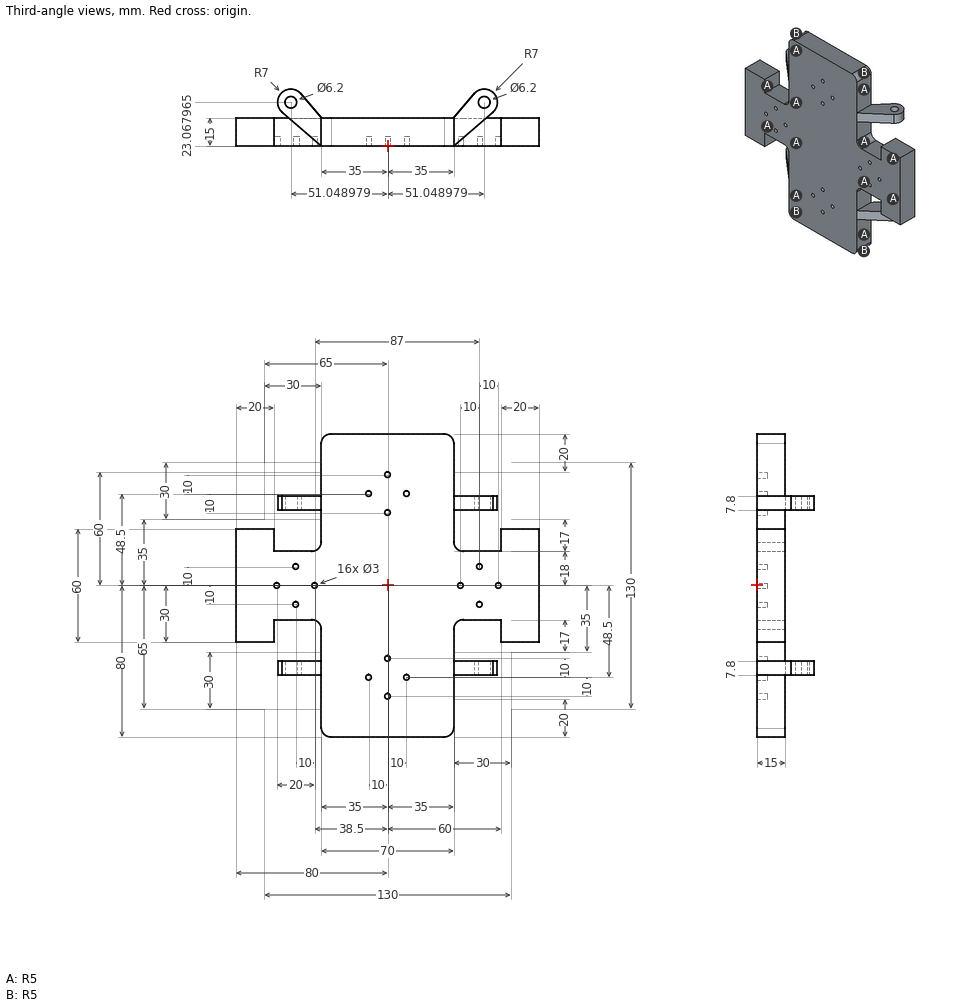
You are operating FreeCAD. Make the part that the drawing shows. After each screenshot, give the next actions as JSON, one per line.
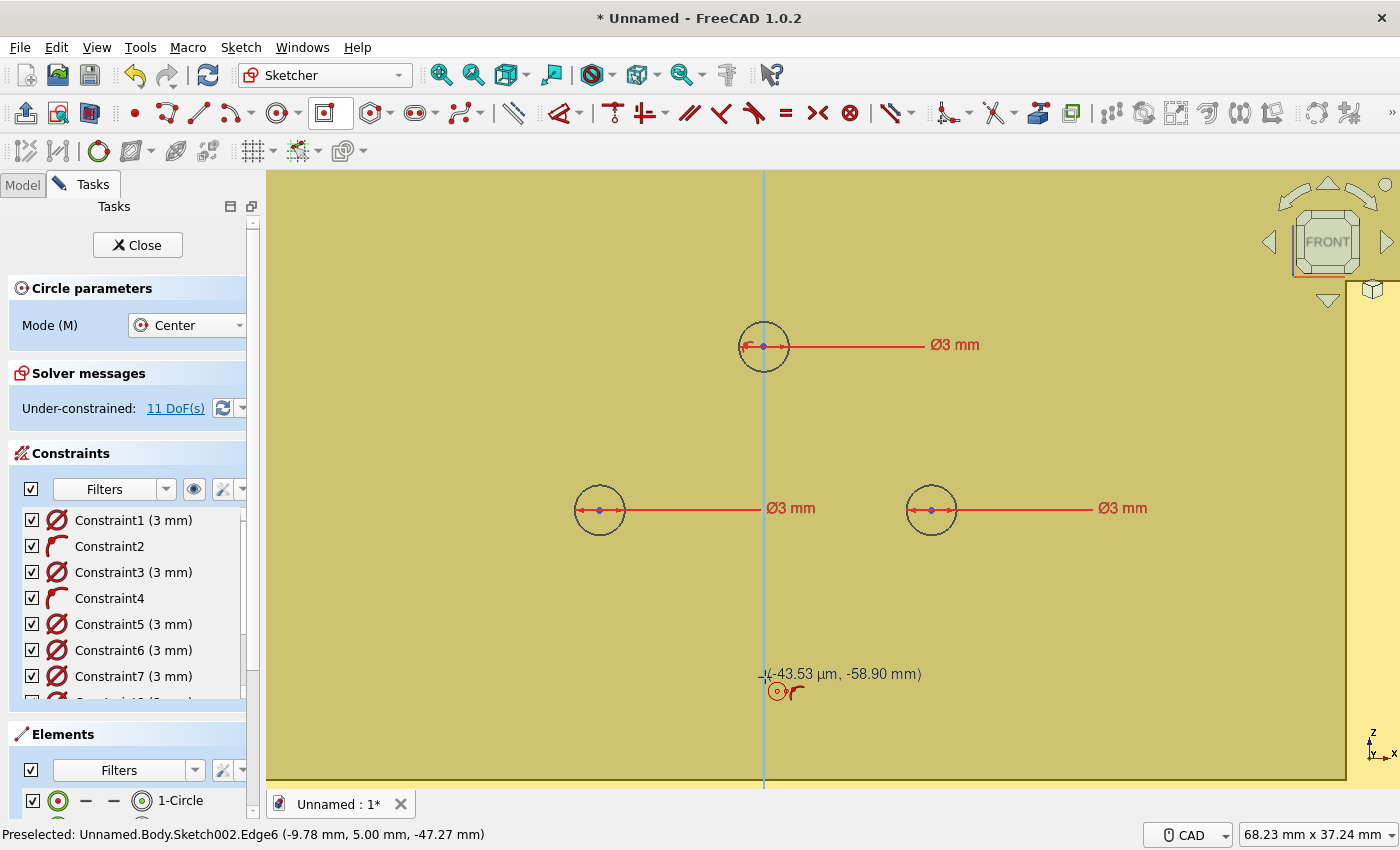
{"action": "scroll", "coordinate": [765, 677], "scroll_direction": "down", "scroll_amount": 8}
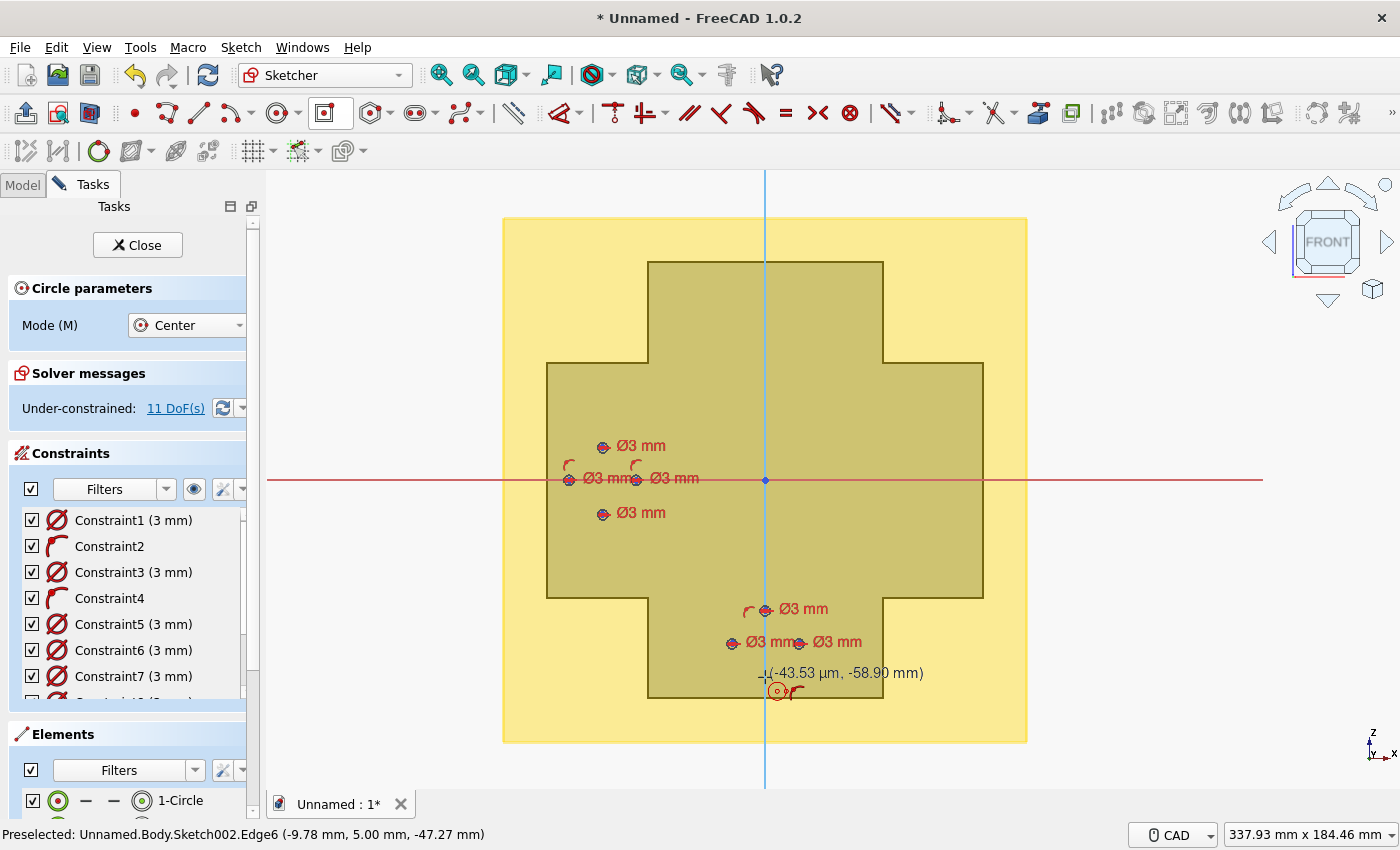
{"action": "left_click", "coordinate": [765, 677]}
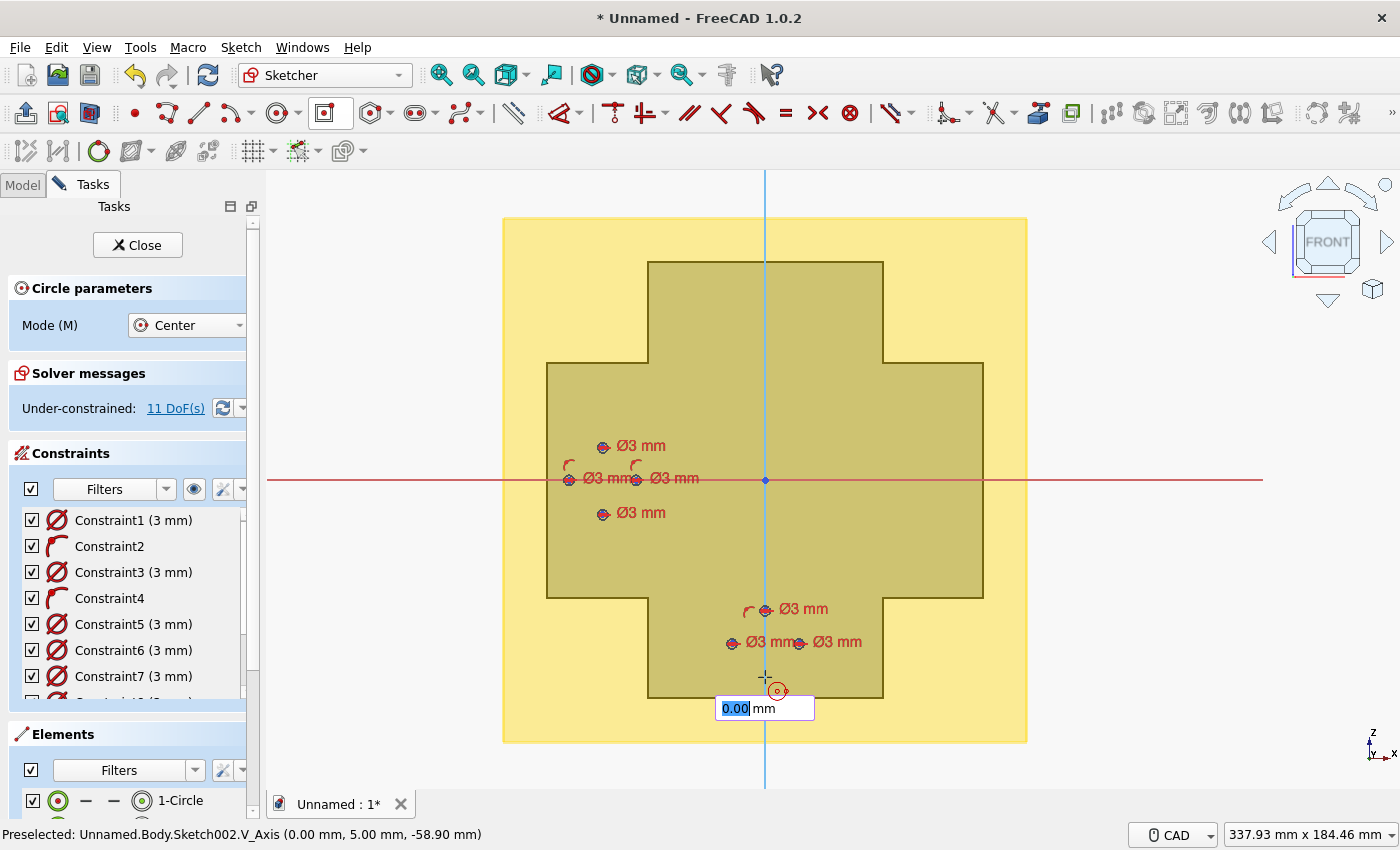
{"action": "scroll", "coordinate": [770, 675], "scroll_direction": "up", "scroll_amount": 7}
{"action": "mouse_move", "coordinate": [768, 672]}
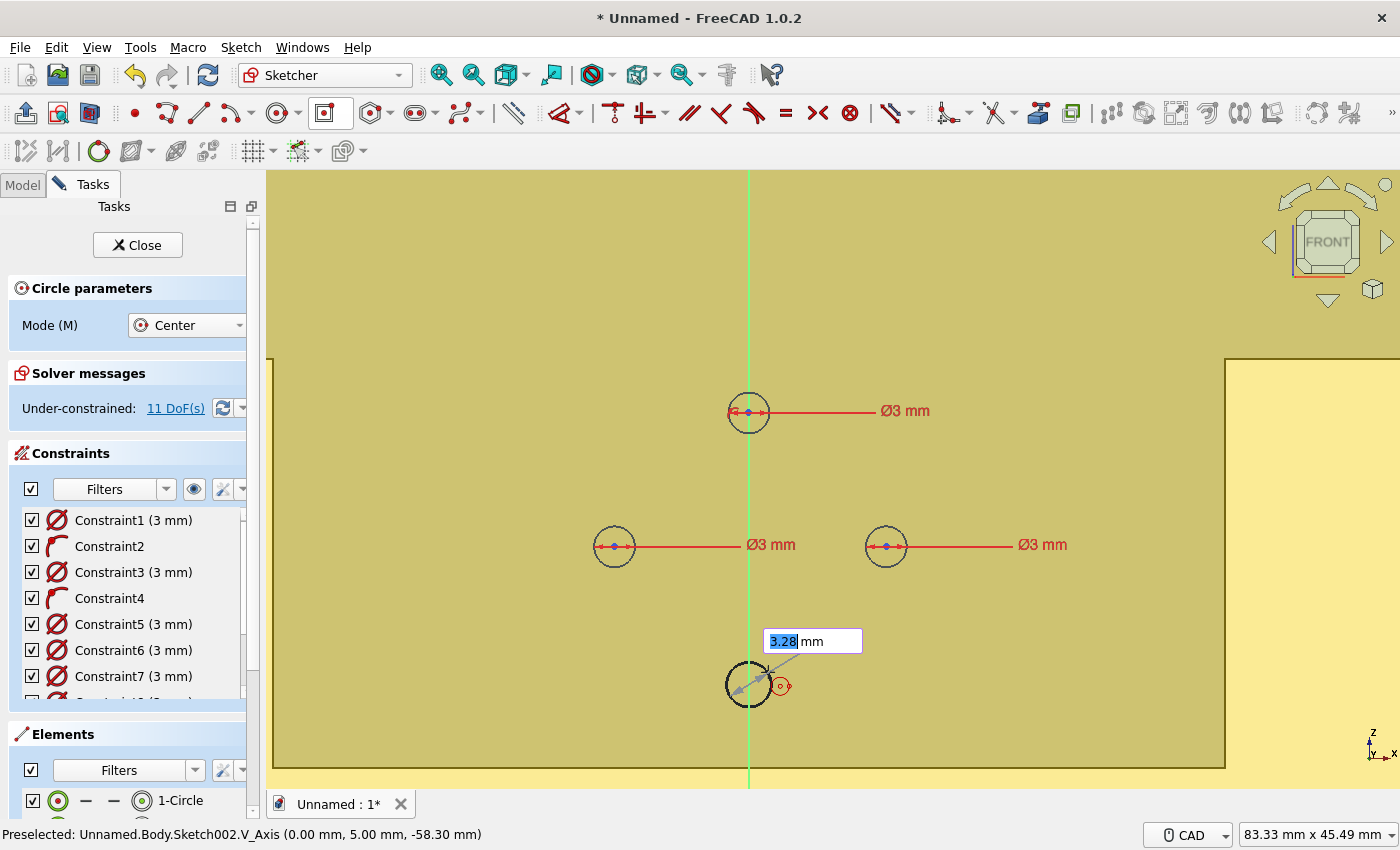
{"action": "type", "text": "3"}
{"action": "key", "text": "Return"}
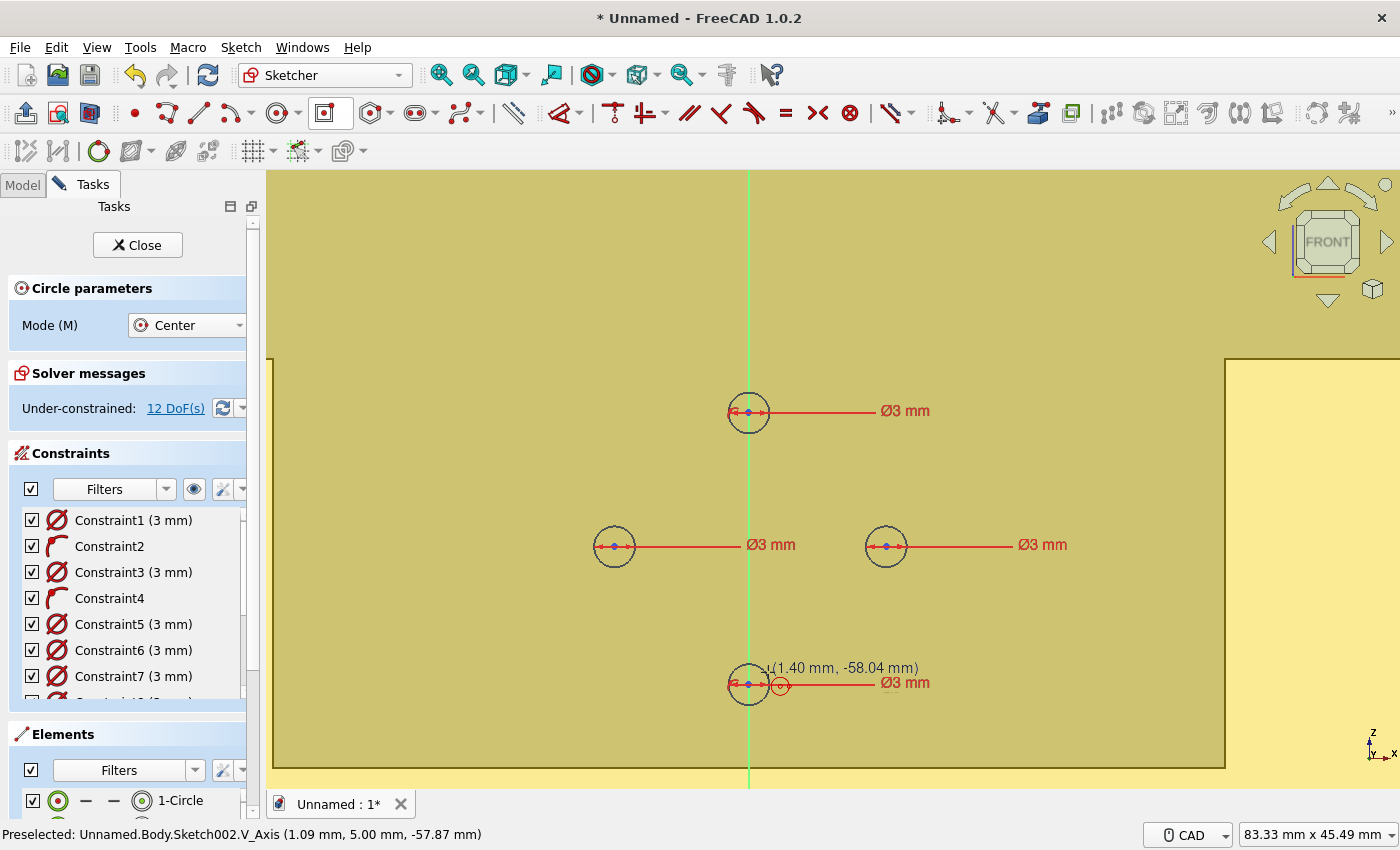
{"action": "scroll", "coordinate": [770, 675], "scroll_direction": "down", "scroll_amount": 7}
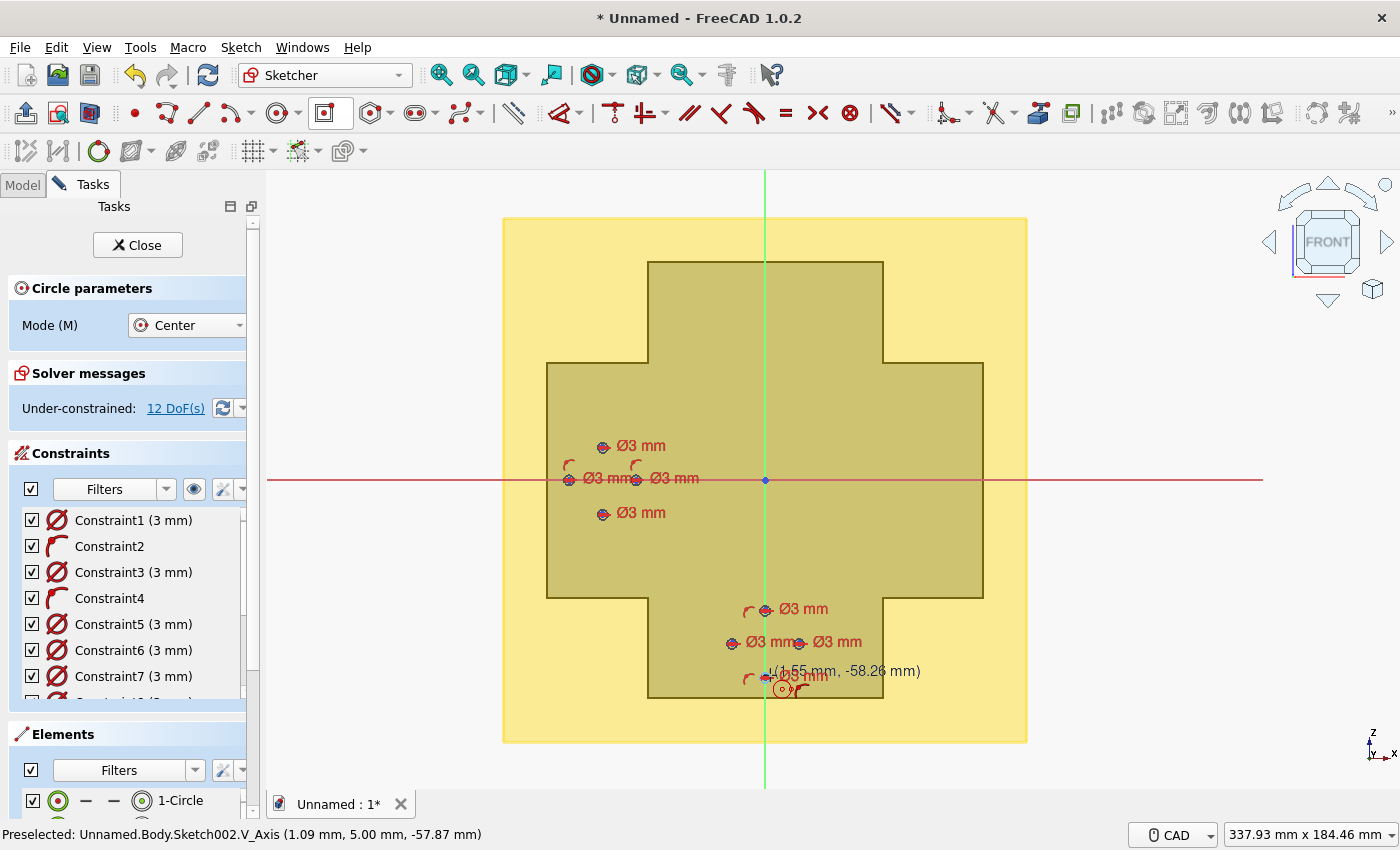
{"action": "scroll", "coordinate": [928, 447], "scroll_direction": "up", "scroll_amount": 8}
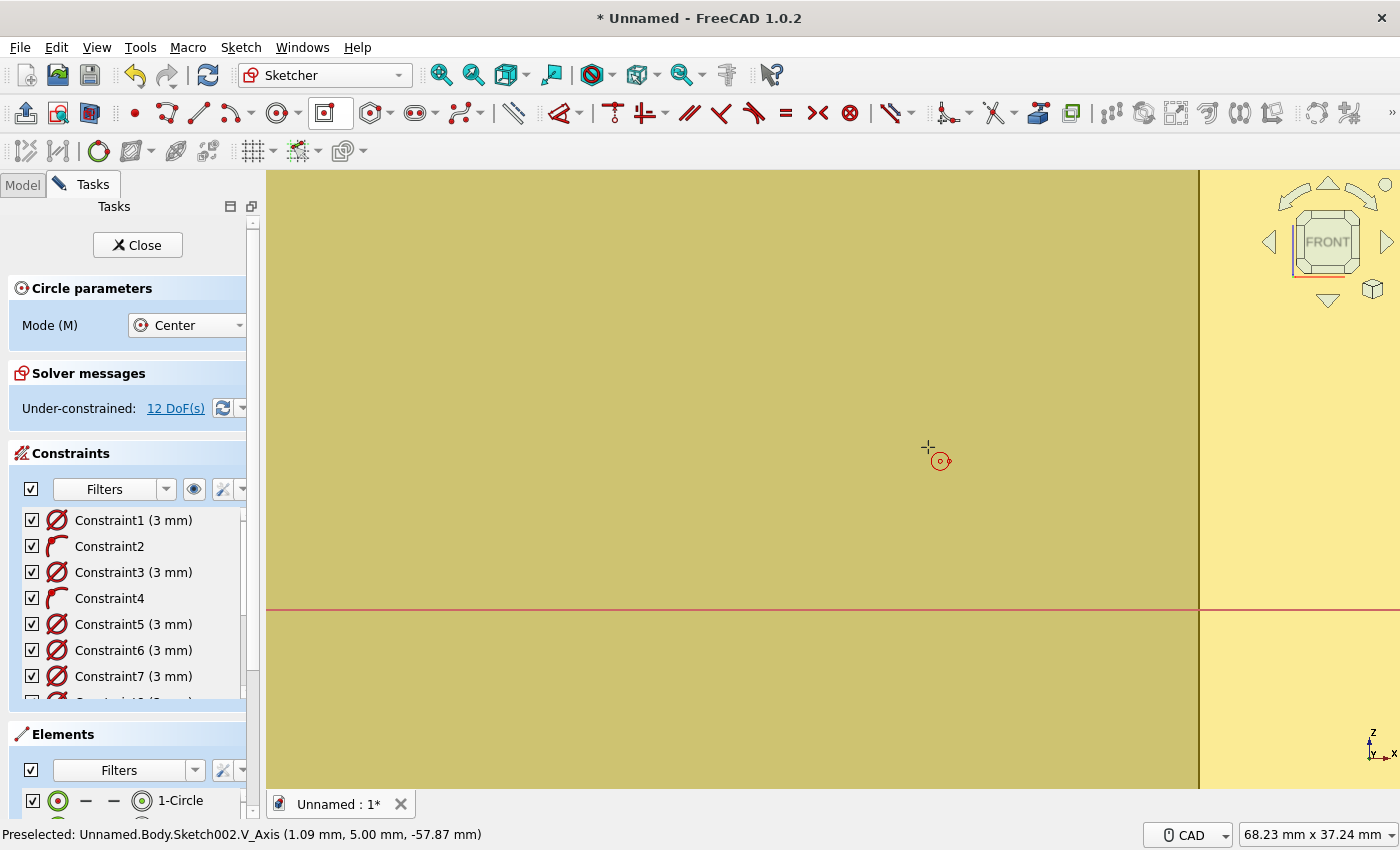
{"action": "scroll", "coordinate": [928, 446], "scroll_direction": "down", "scroll_amount": 8}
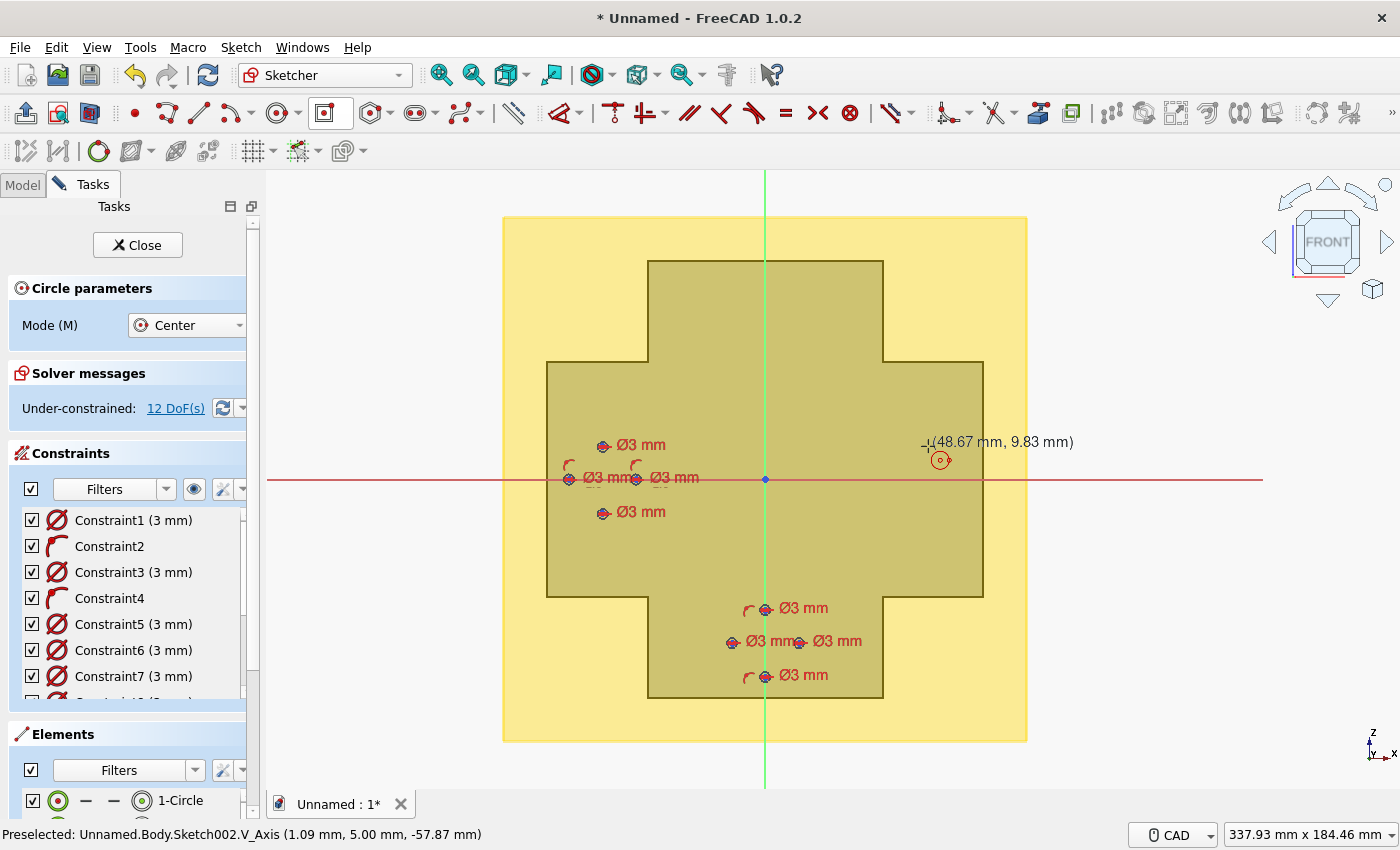
{"action": "left_click", "coordinate": [928, 446]}
{"action": "mouse_move", "coordinate": [931, 442]}